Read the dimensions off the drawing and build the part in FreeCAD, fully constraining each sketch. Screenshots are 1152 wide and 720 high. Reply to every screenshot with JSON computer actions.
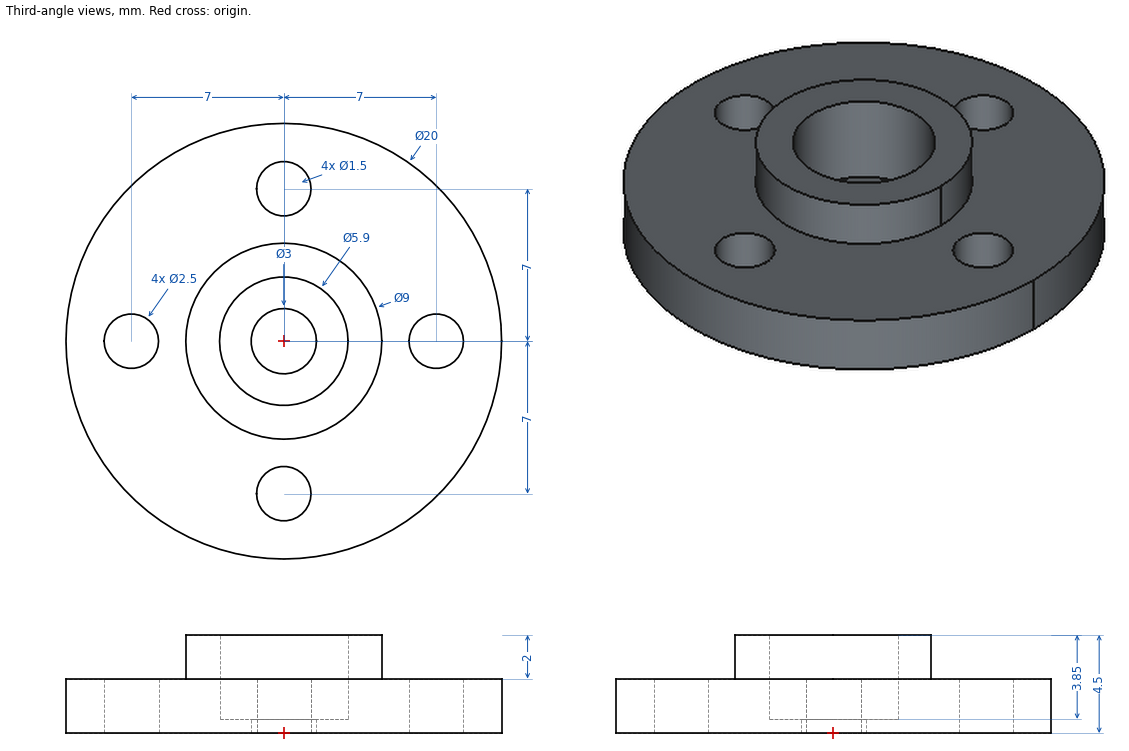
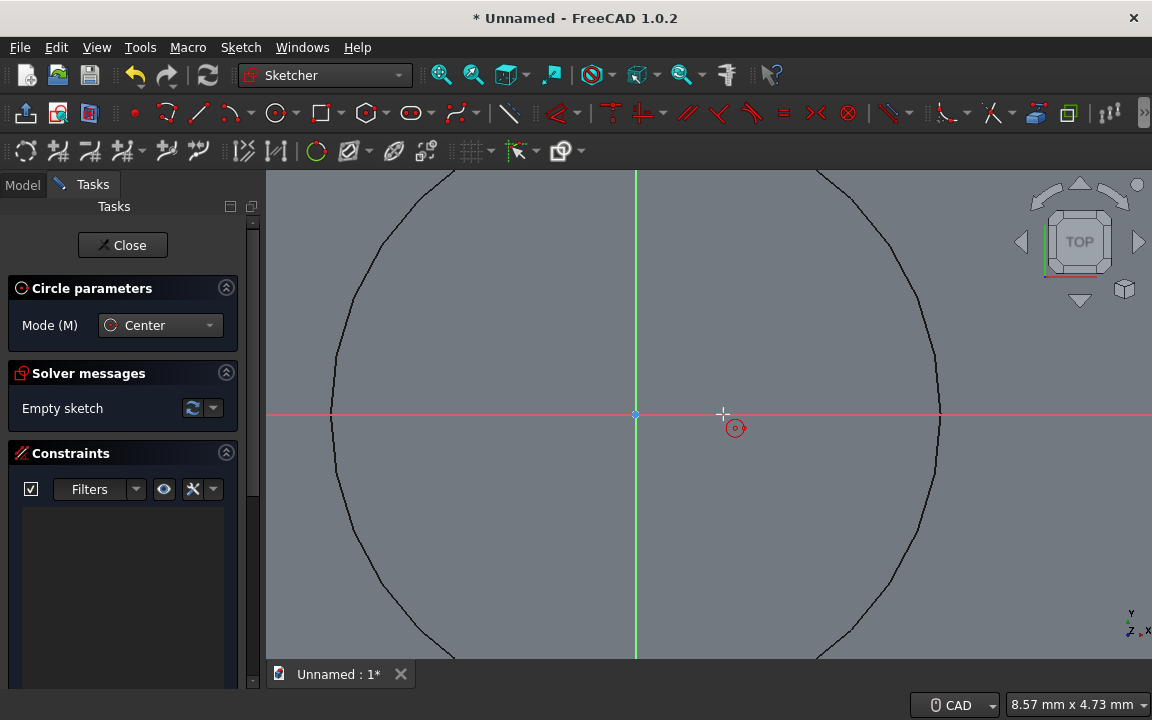
{"action": "left_click", "coordinate": [636, 414]}
{"action": "left_click", "coordinate": [745, 305]}
{"action": "key", "text": "Escape"}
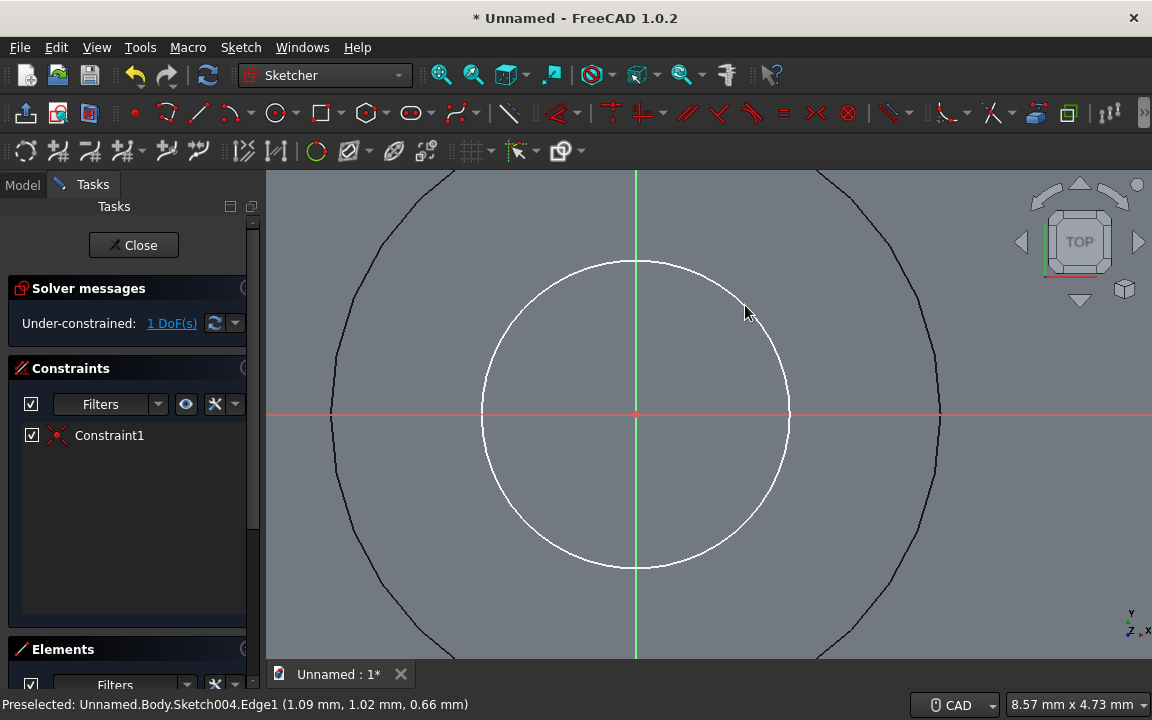
{"action": "key", "text": "d"}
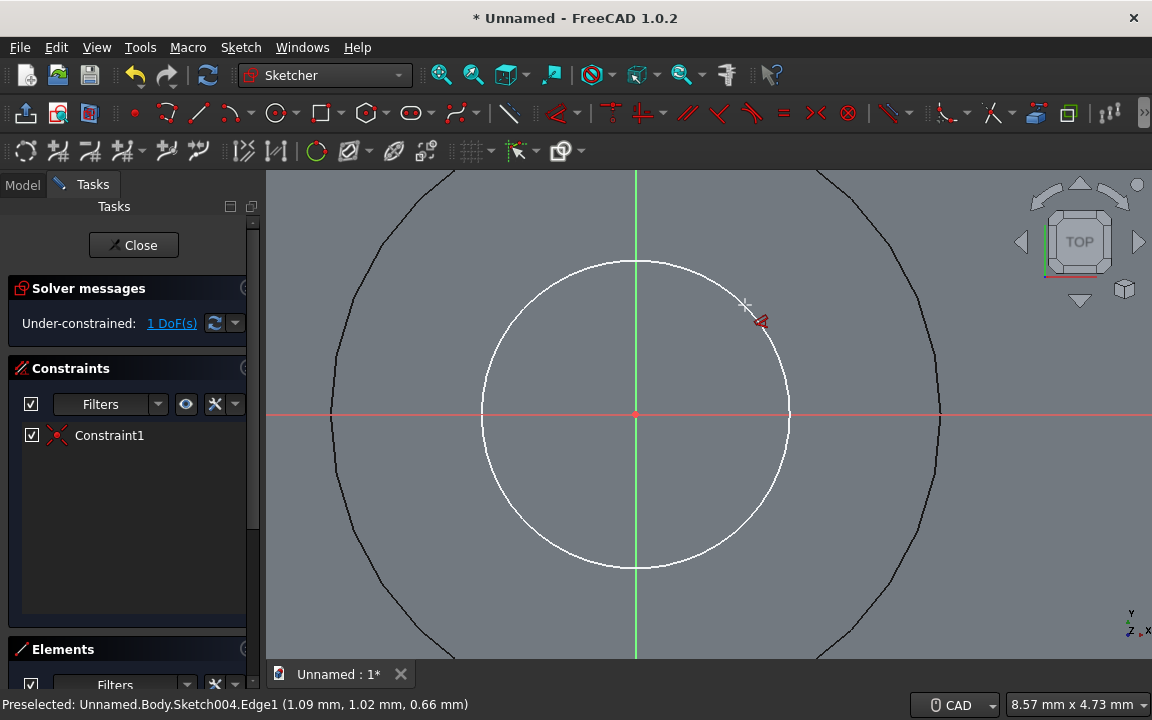
{"action": "left_click", "coordinate": [744, 305]}
{"action": "left_click", "coordinate": [767, 282]}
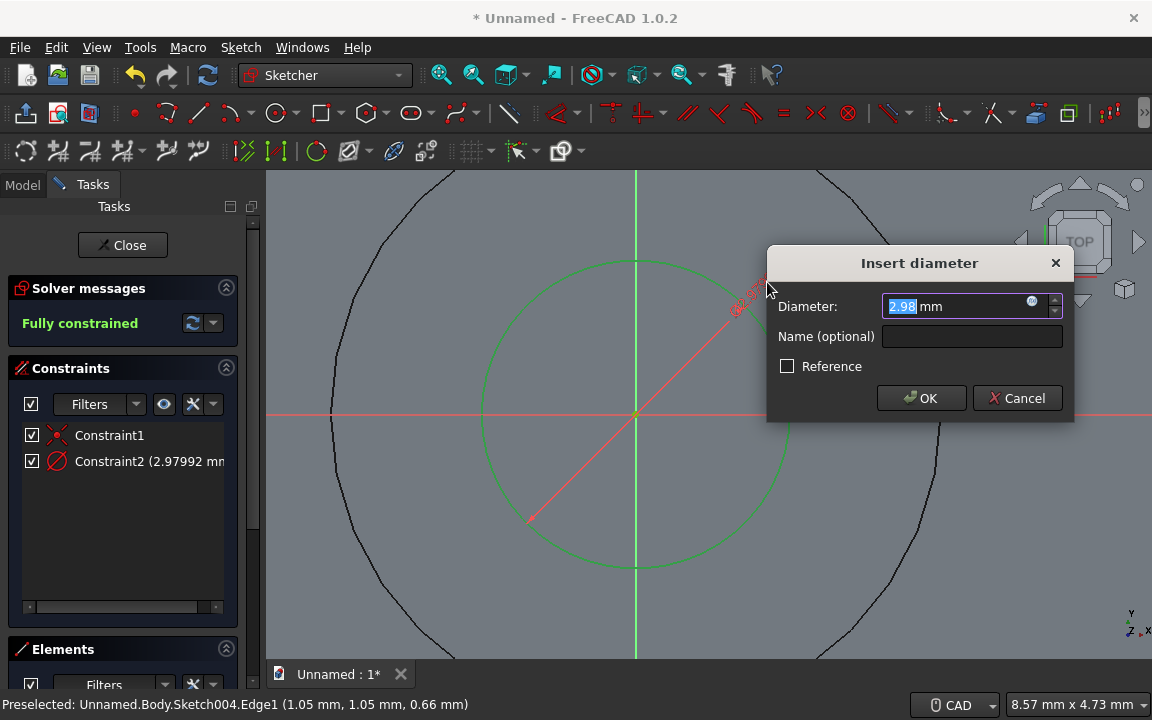
{"action": "type", "text": "3"}
{"action": "key", "text": "Return"}
{"action": "key", "text": "Escape"}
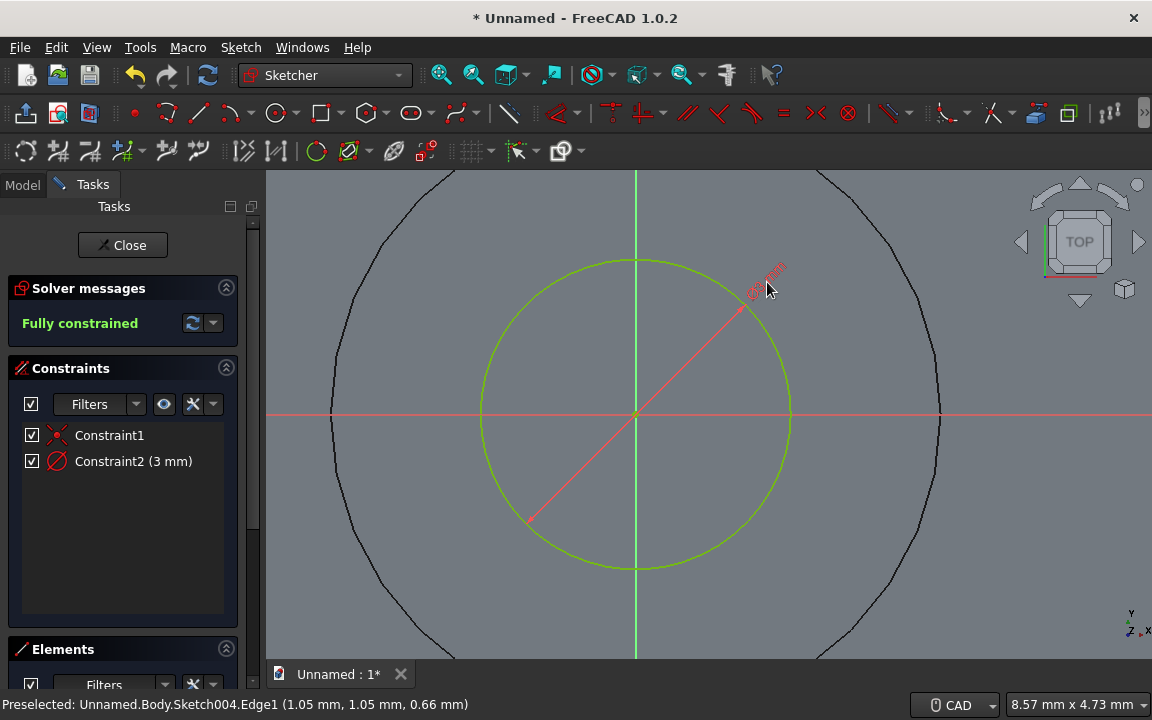
{"action": "left_click", "coordinate": [123, 245]}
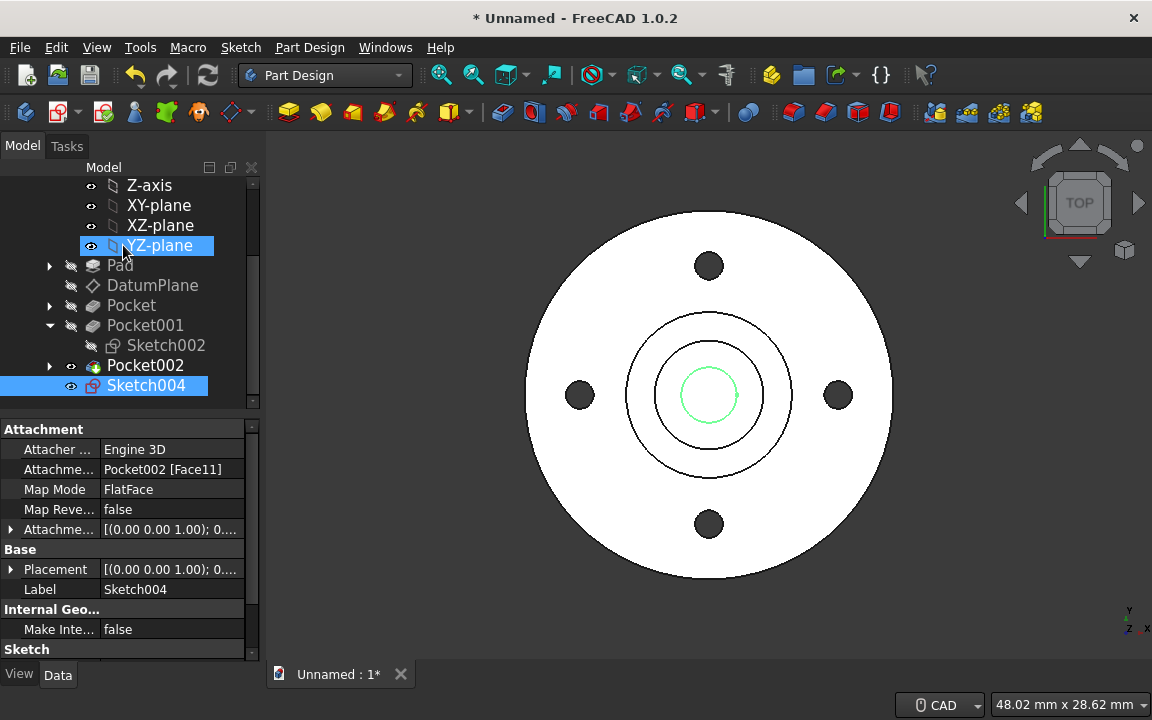
{"action": "left_click", "coordinate": [504, 112]}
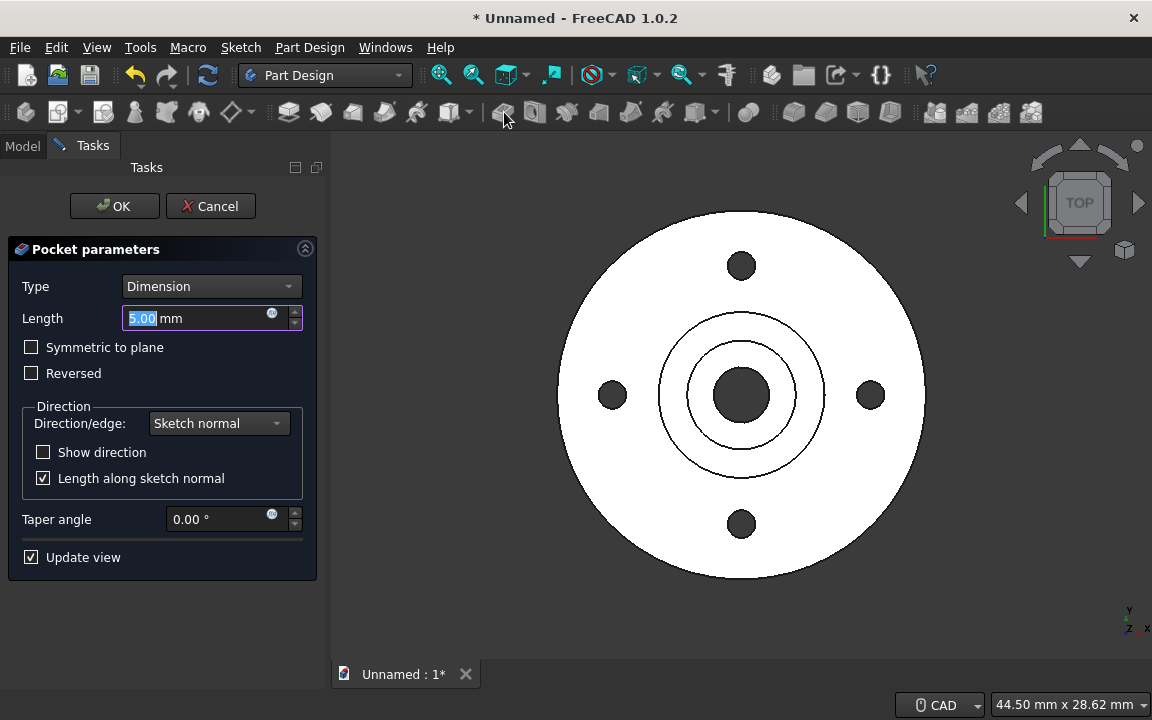
{"action": "left_click", "coordinate": [212, 286]}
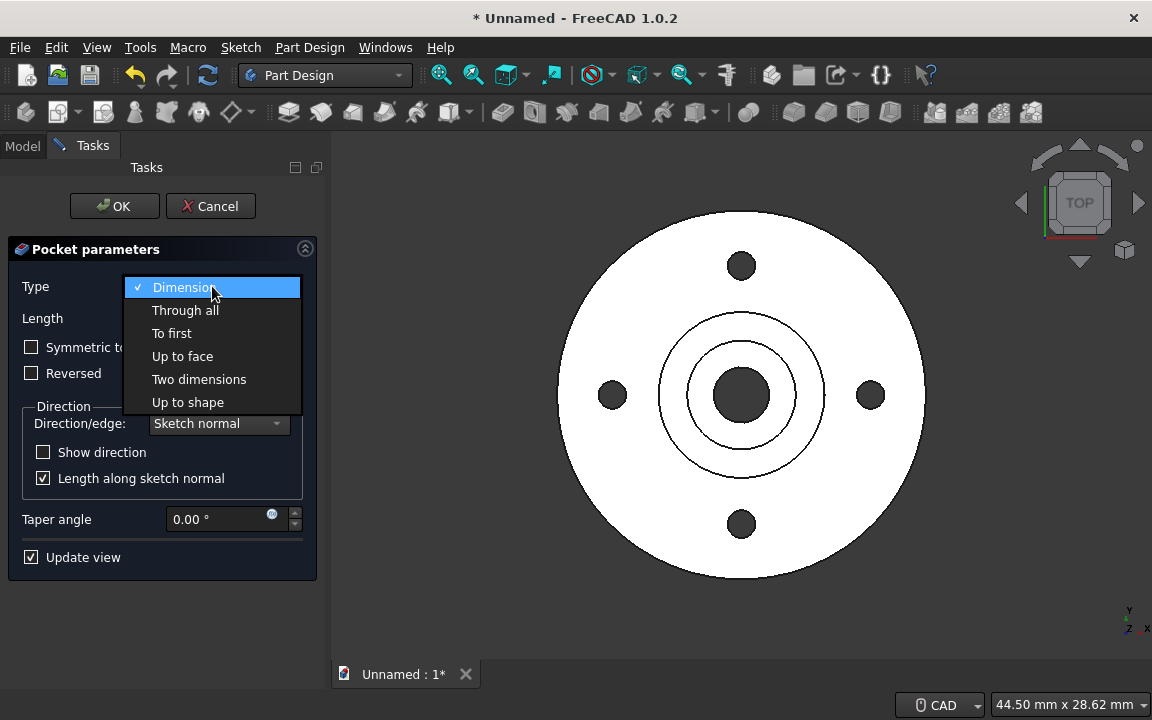
{"action": "left_click", "coordinate": [212, 310]}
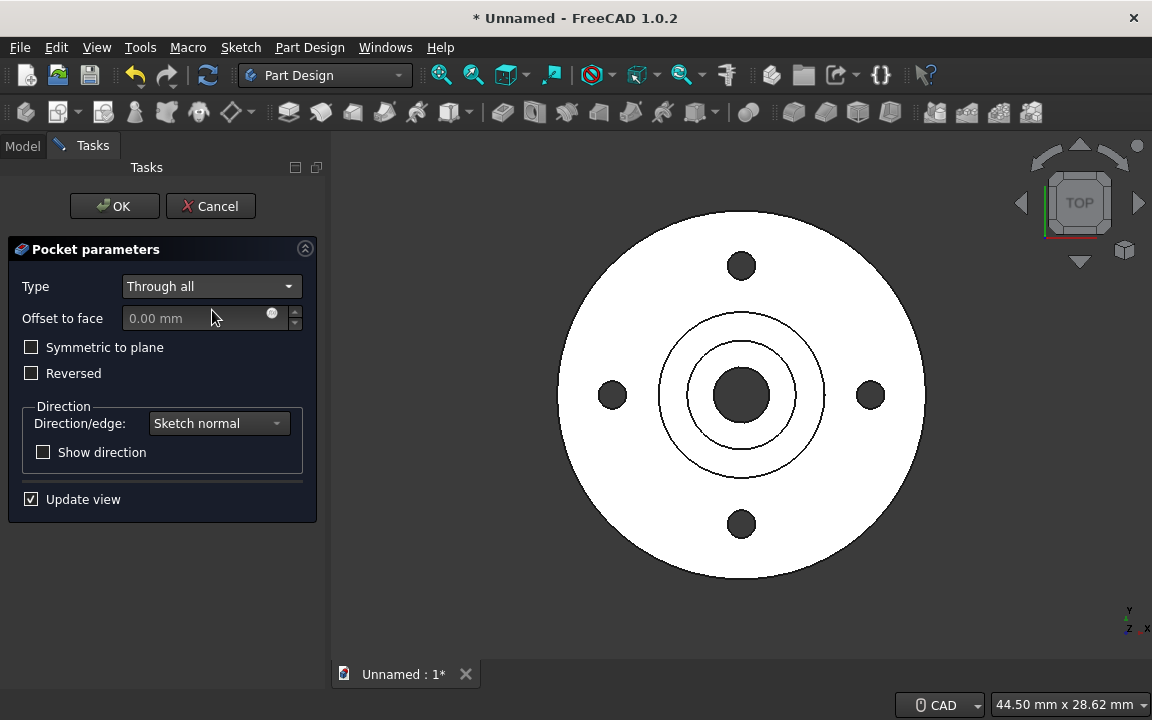
{"action": "left_click", "coordinate": [115, 206]}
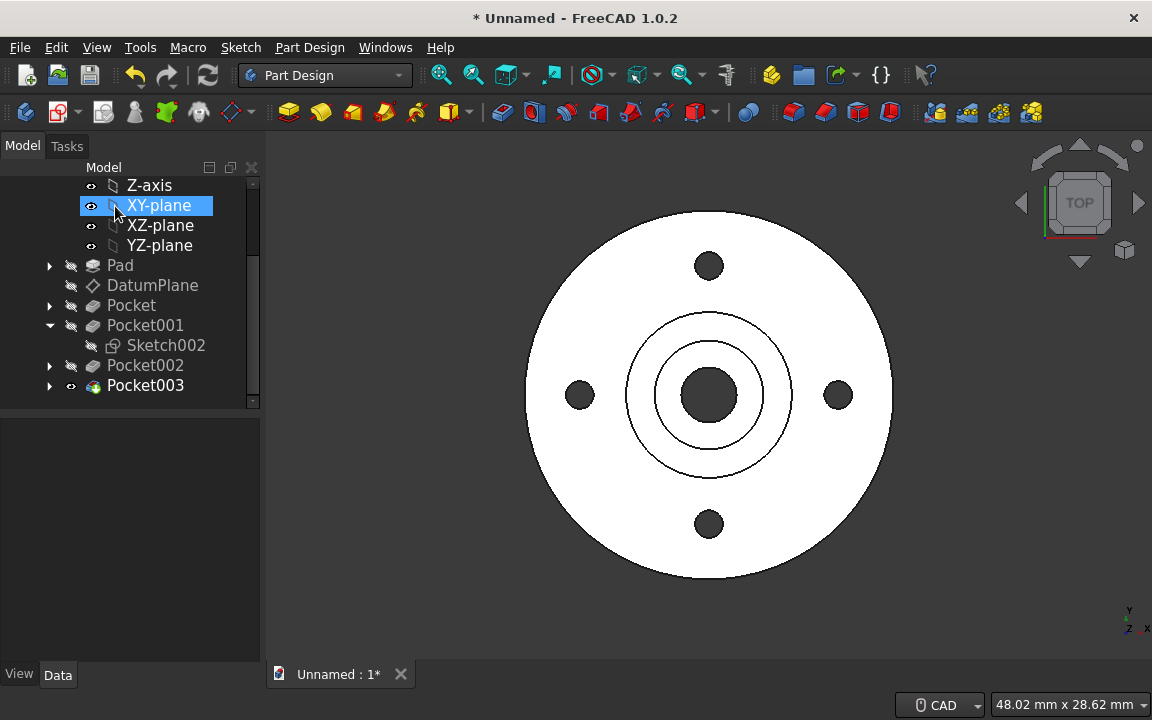
{"action": "left_click", "coordinate": [814, 499]}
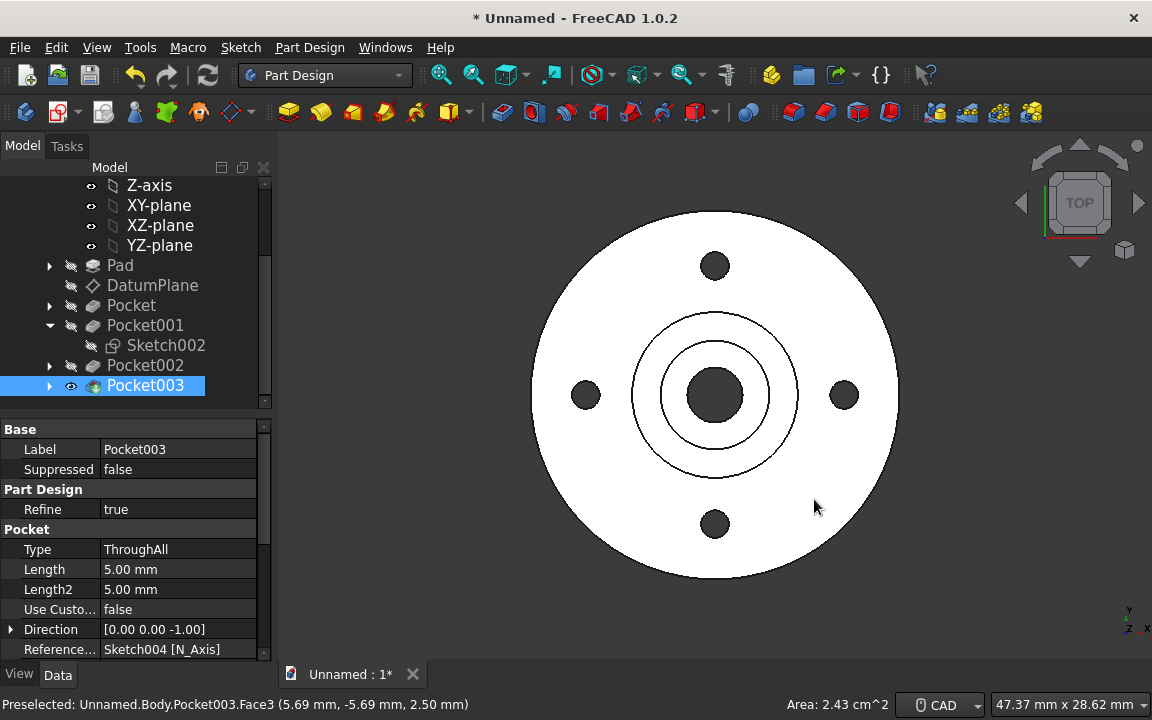
{"action": "left_click", "coordinate": [58, 112]}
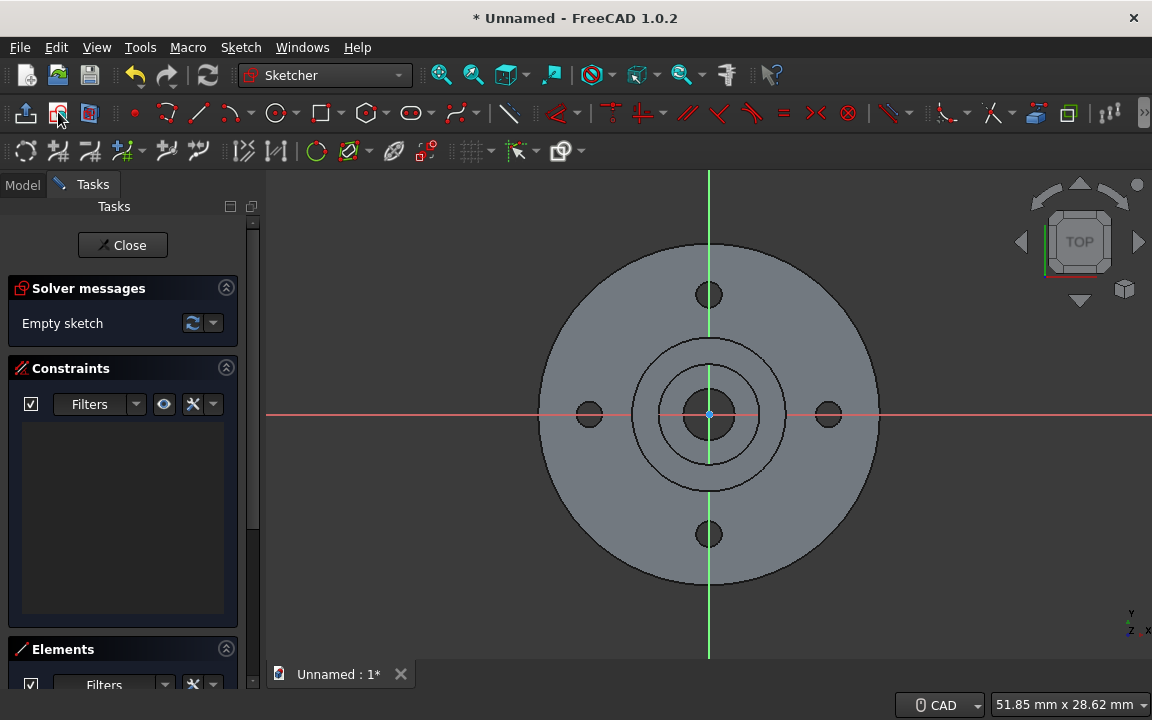
{"action": "left_click", "coordinate": [90, 114]}